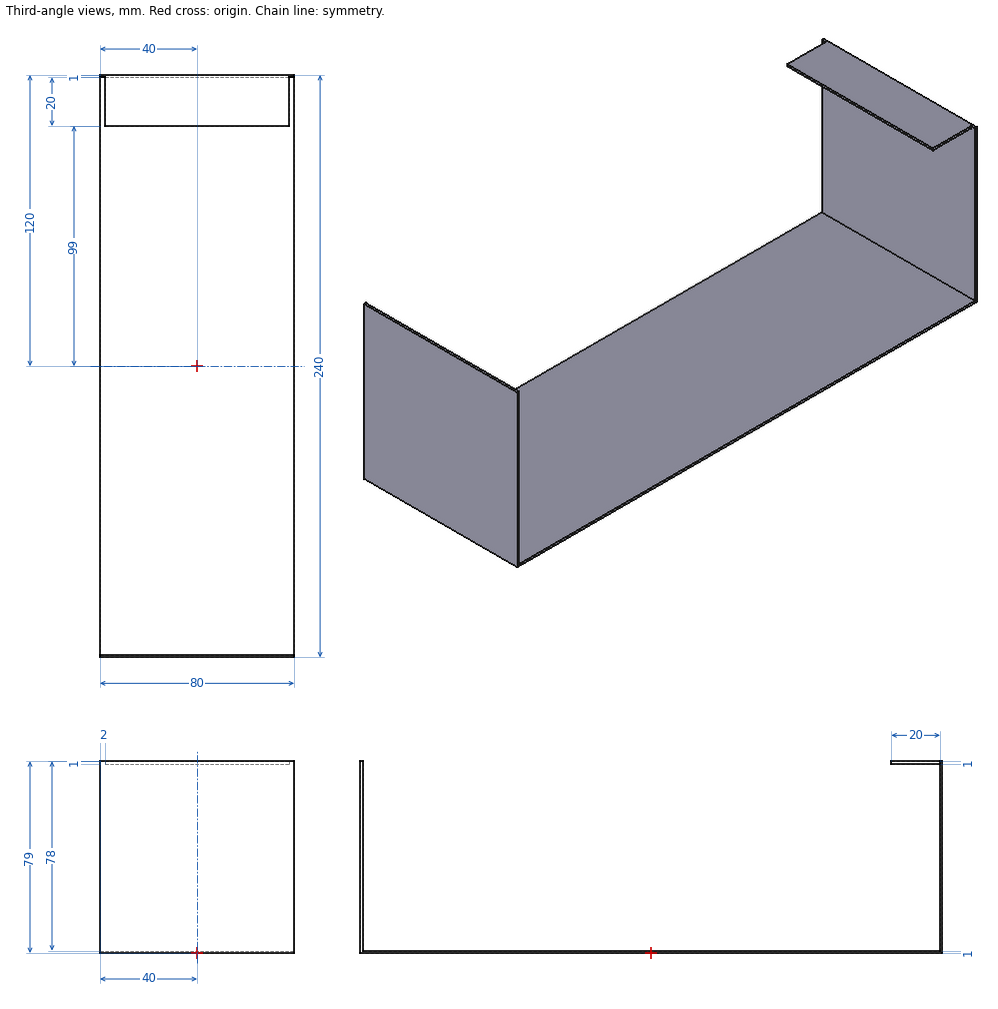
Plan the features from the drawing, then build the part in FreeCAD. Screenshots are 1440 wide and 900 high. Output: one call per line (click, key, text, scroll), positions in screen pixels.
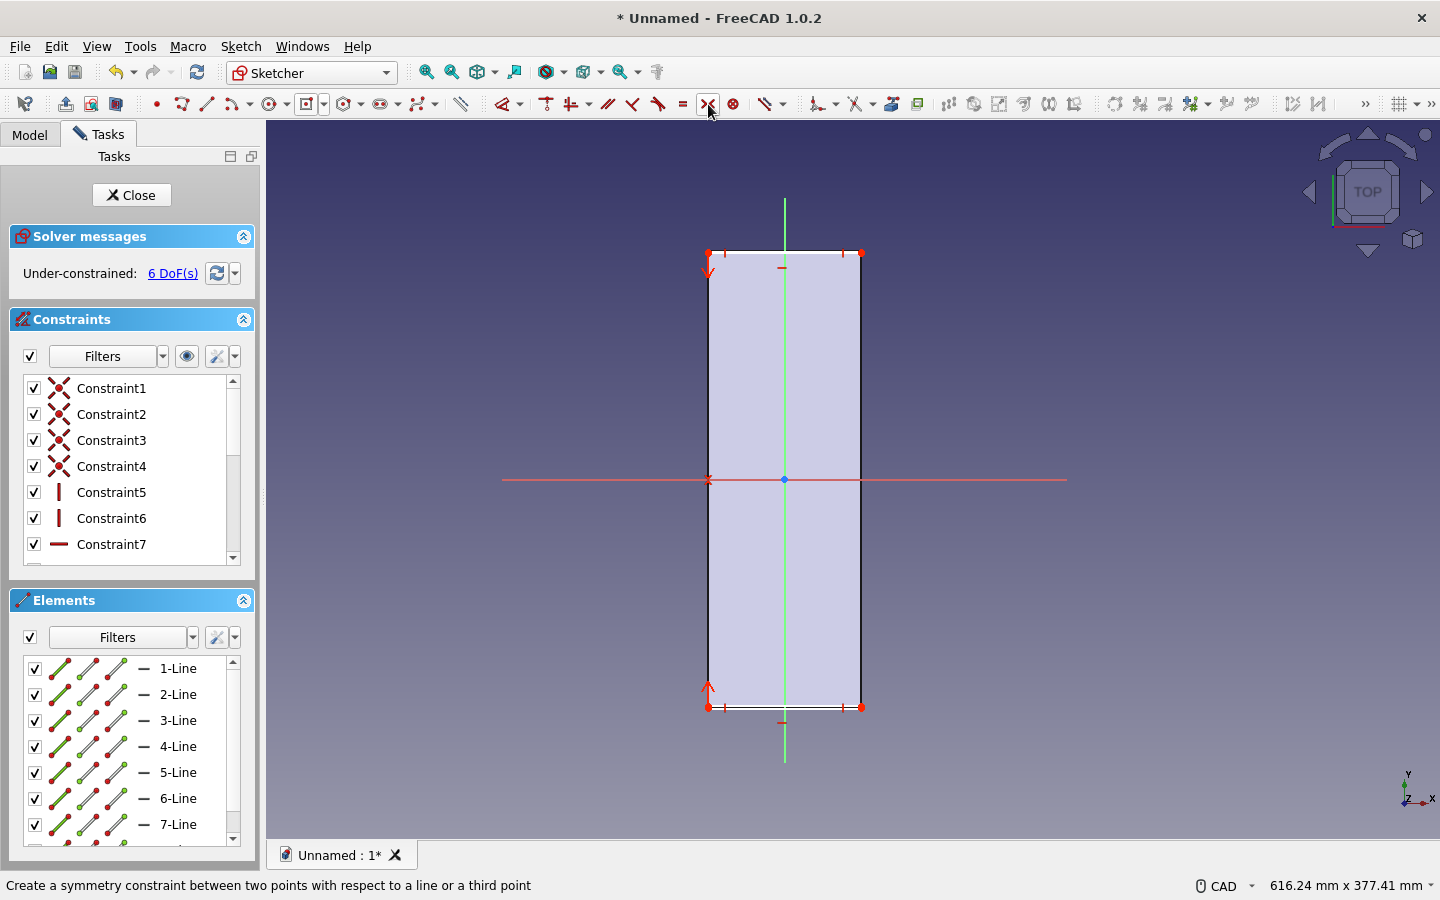
scroll(861, 252, up, 11)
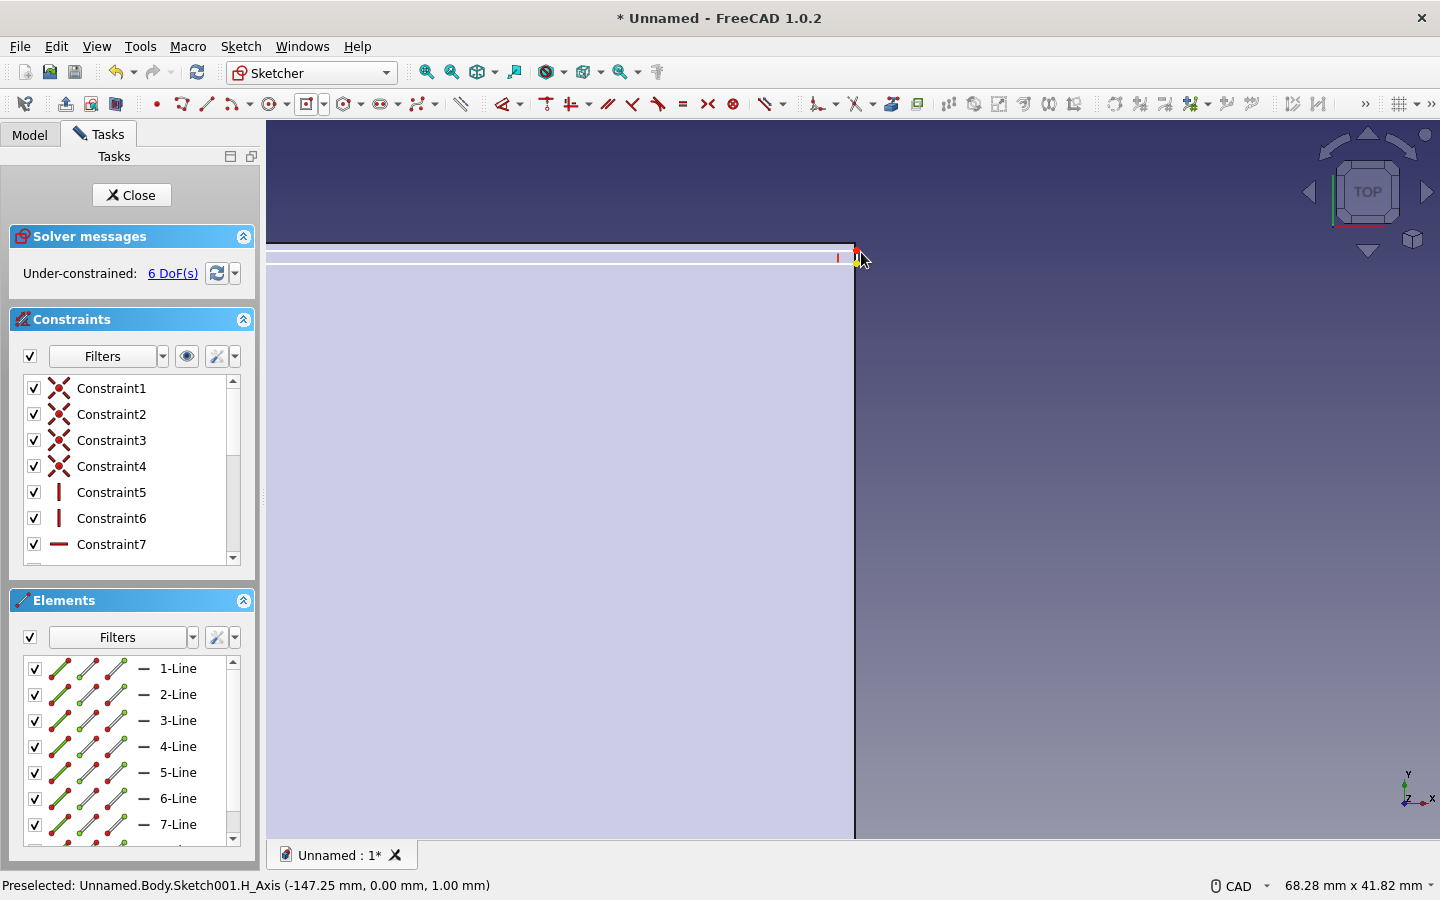
click(857, 251)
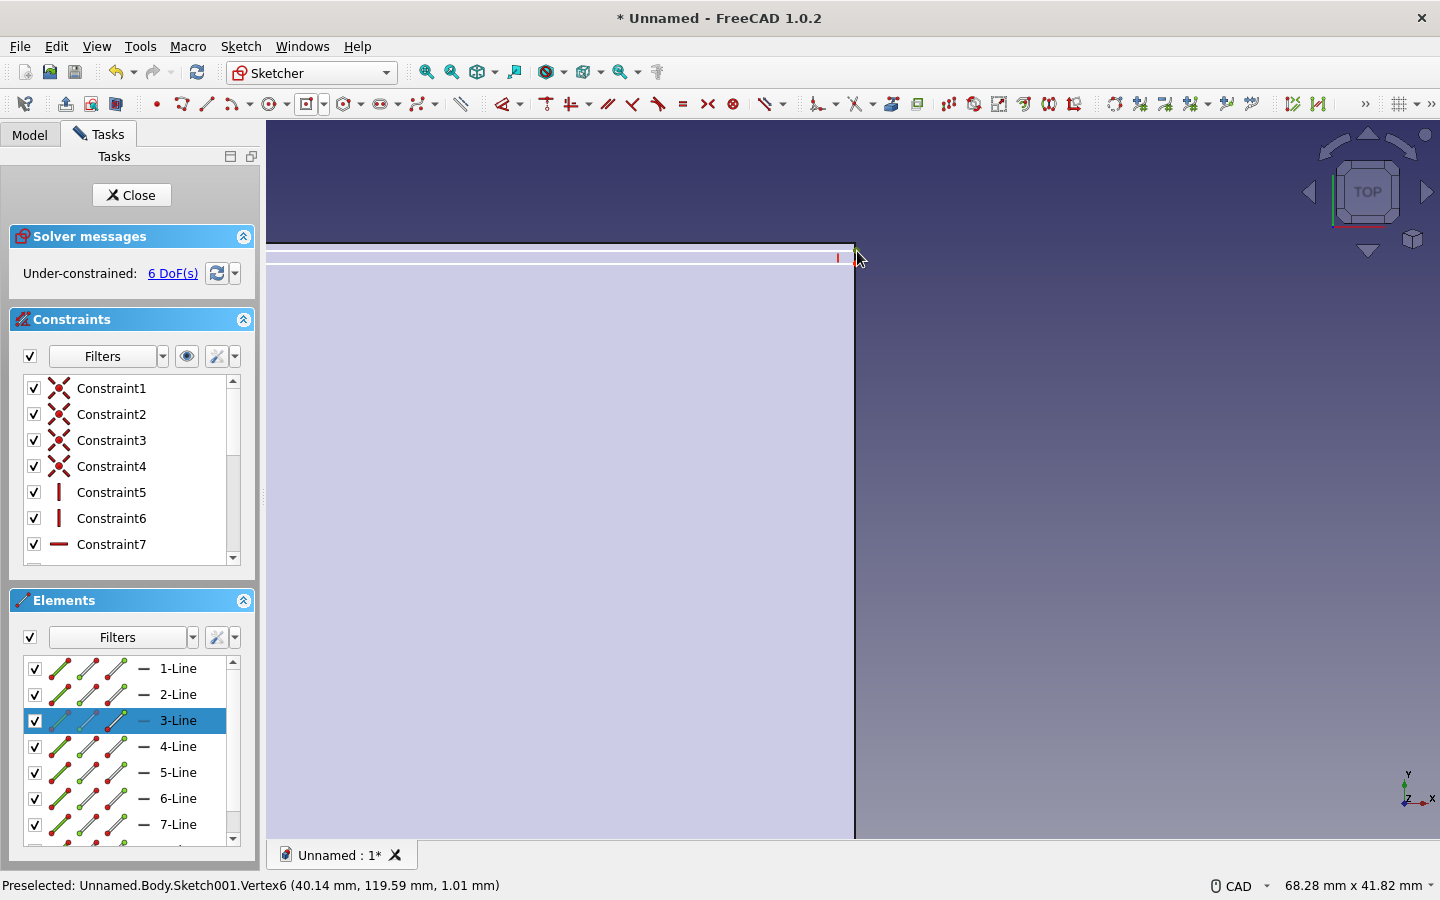
scroll(861, 252, down, 11)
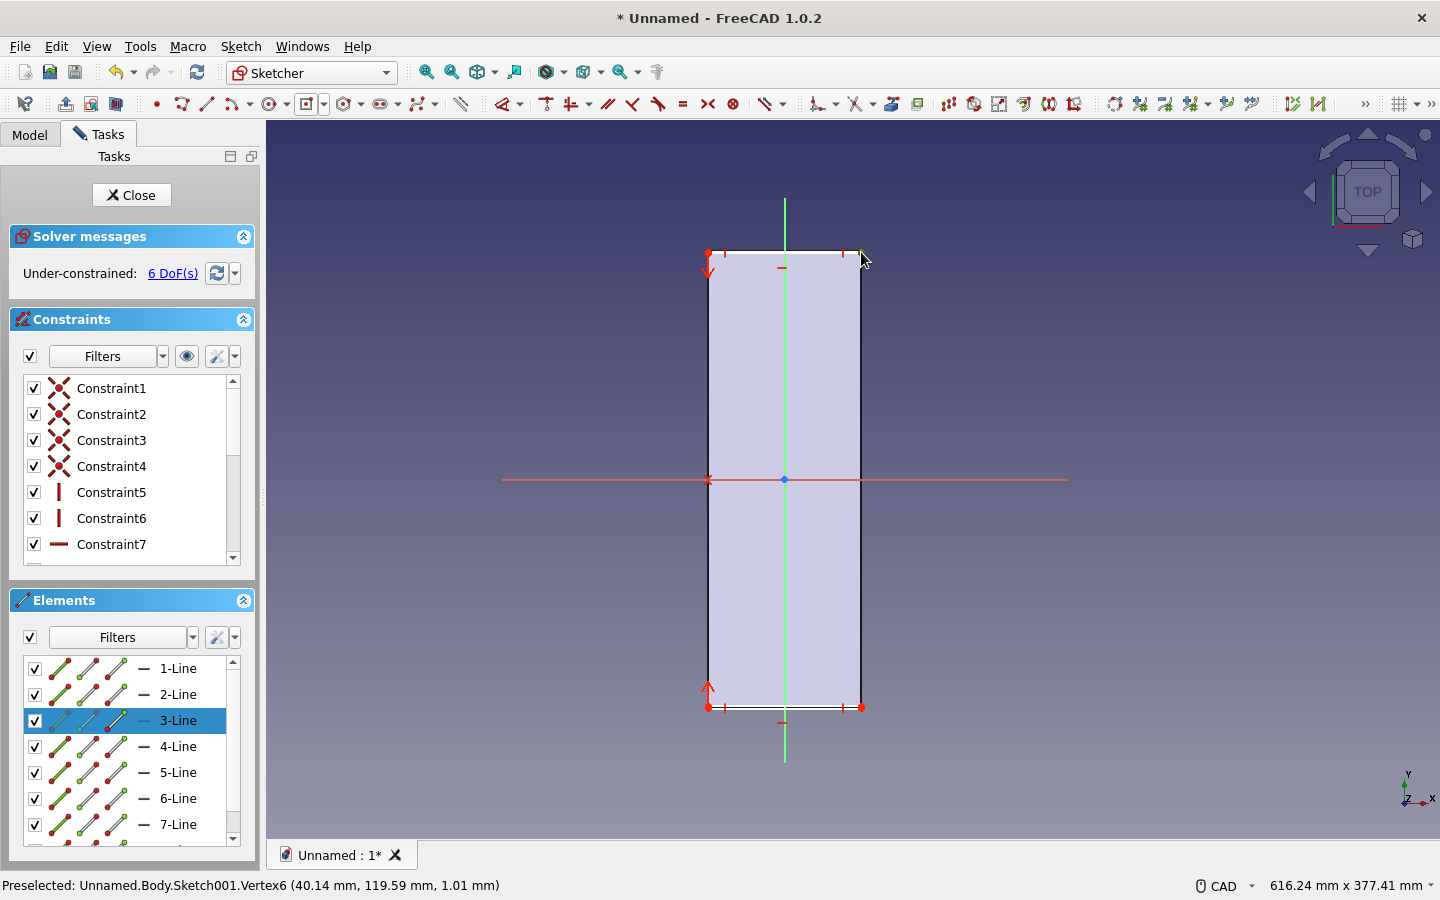
scroll(861, 709, up, 8)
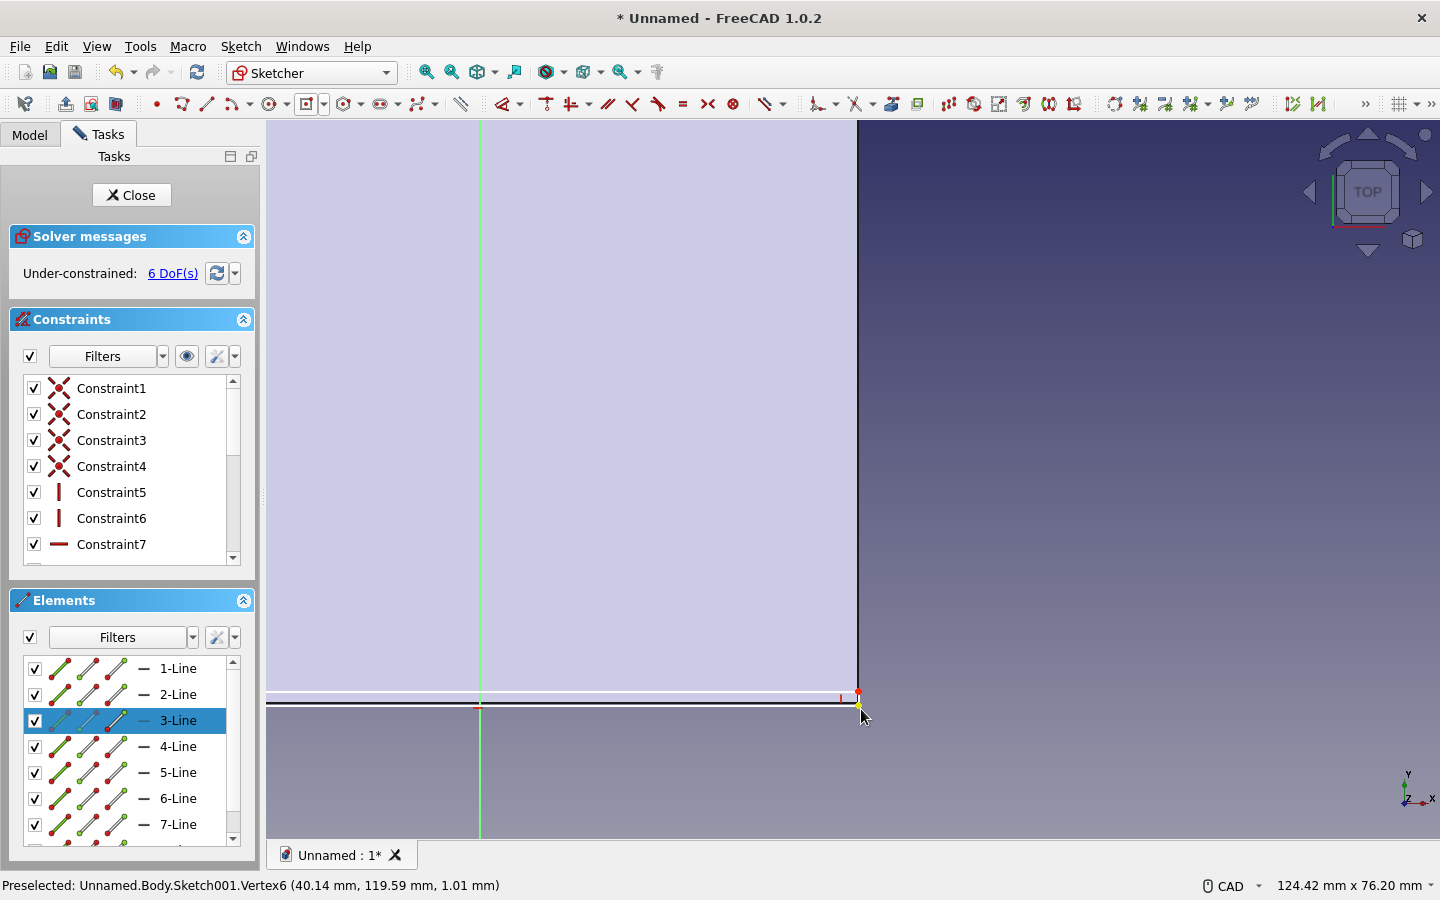
click(859, 706)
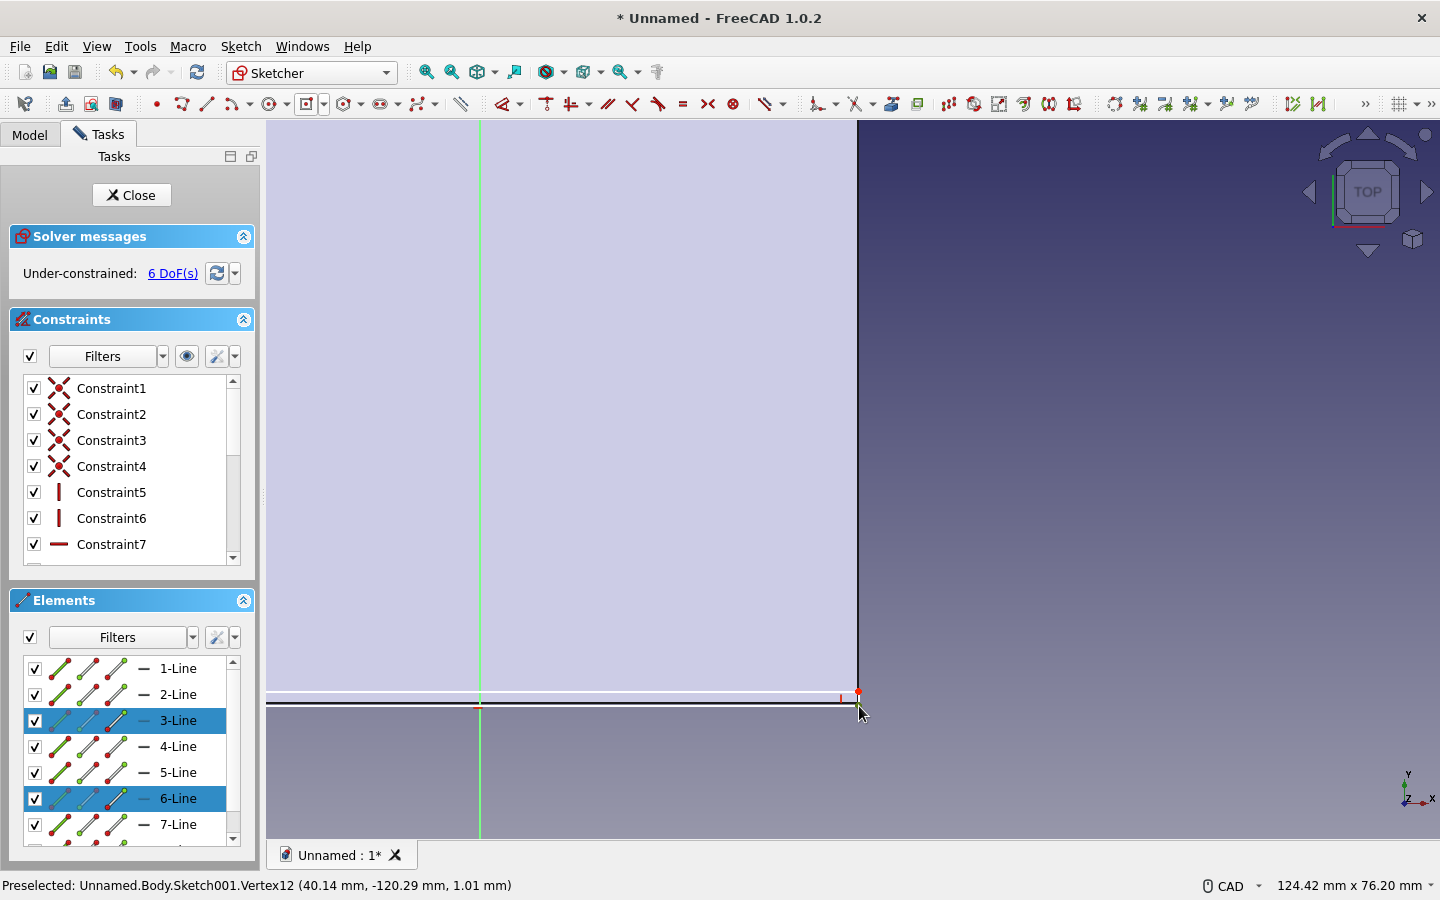
scroll(861, 709, down, 8)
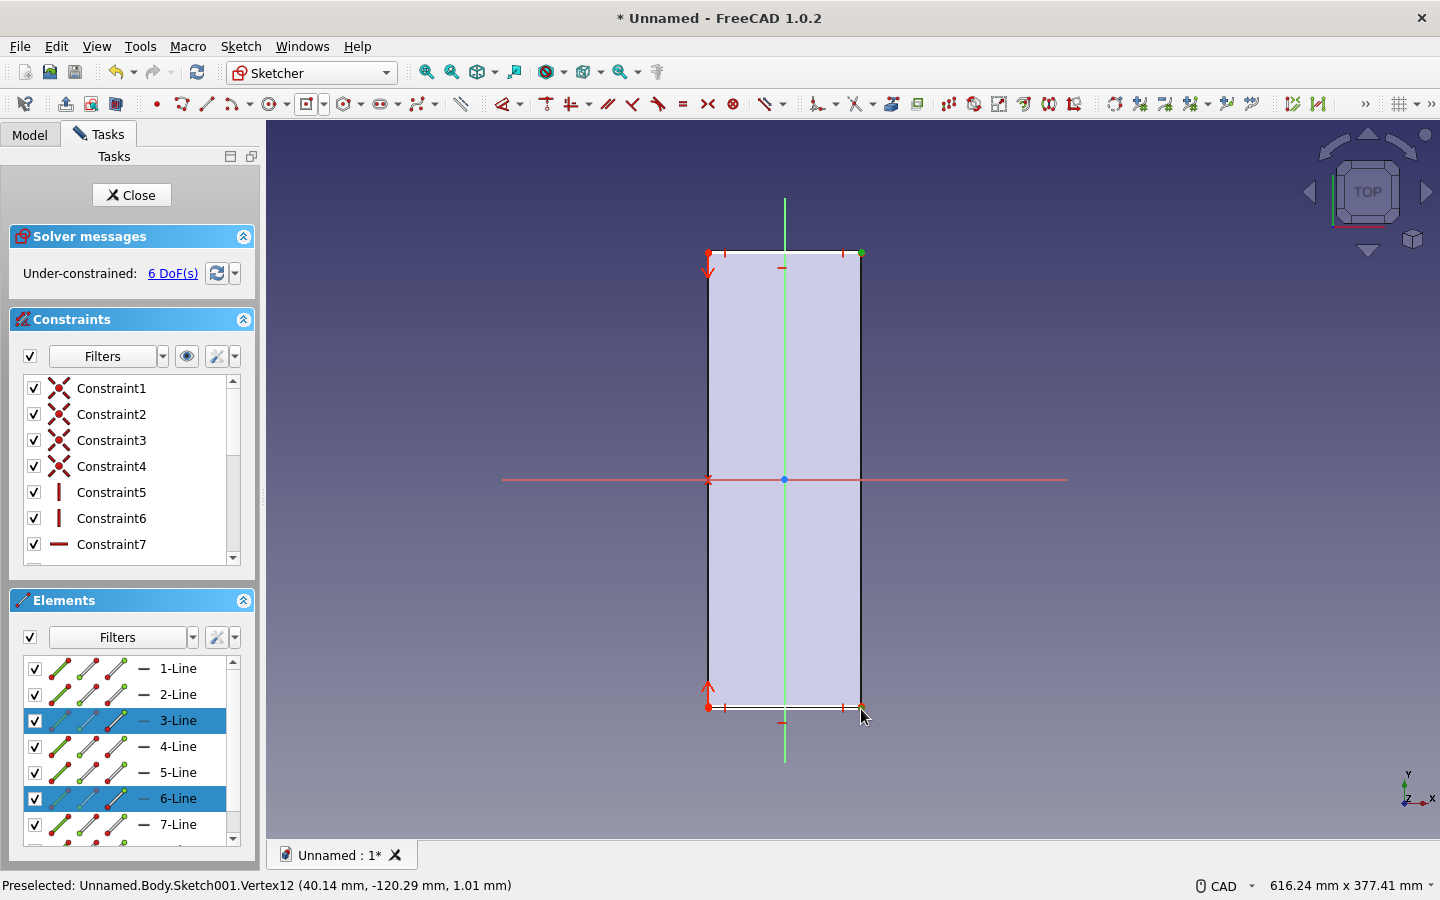
click(504, 480)